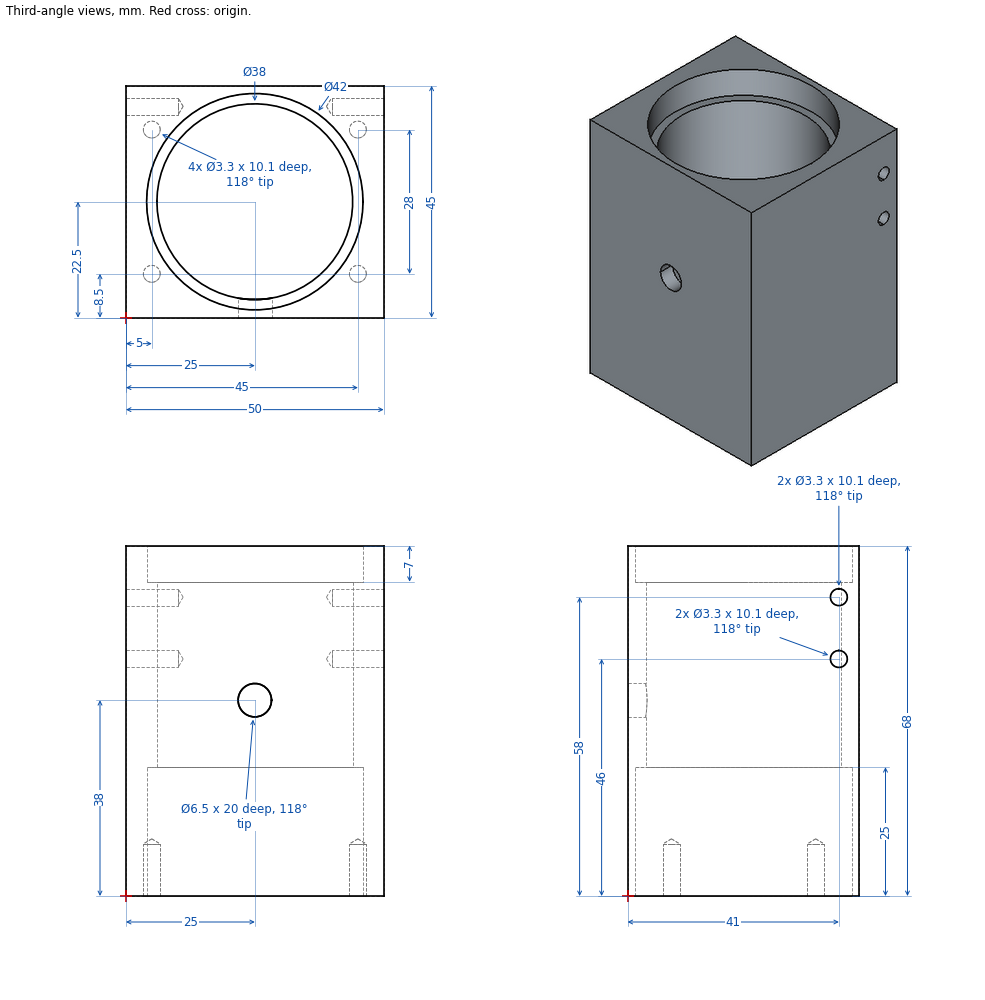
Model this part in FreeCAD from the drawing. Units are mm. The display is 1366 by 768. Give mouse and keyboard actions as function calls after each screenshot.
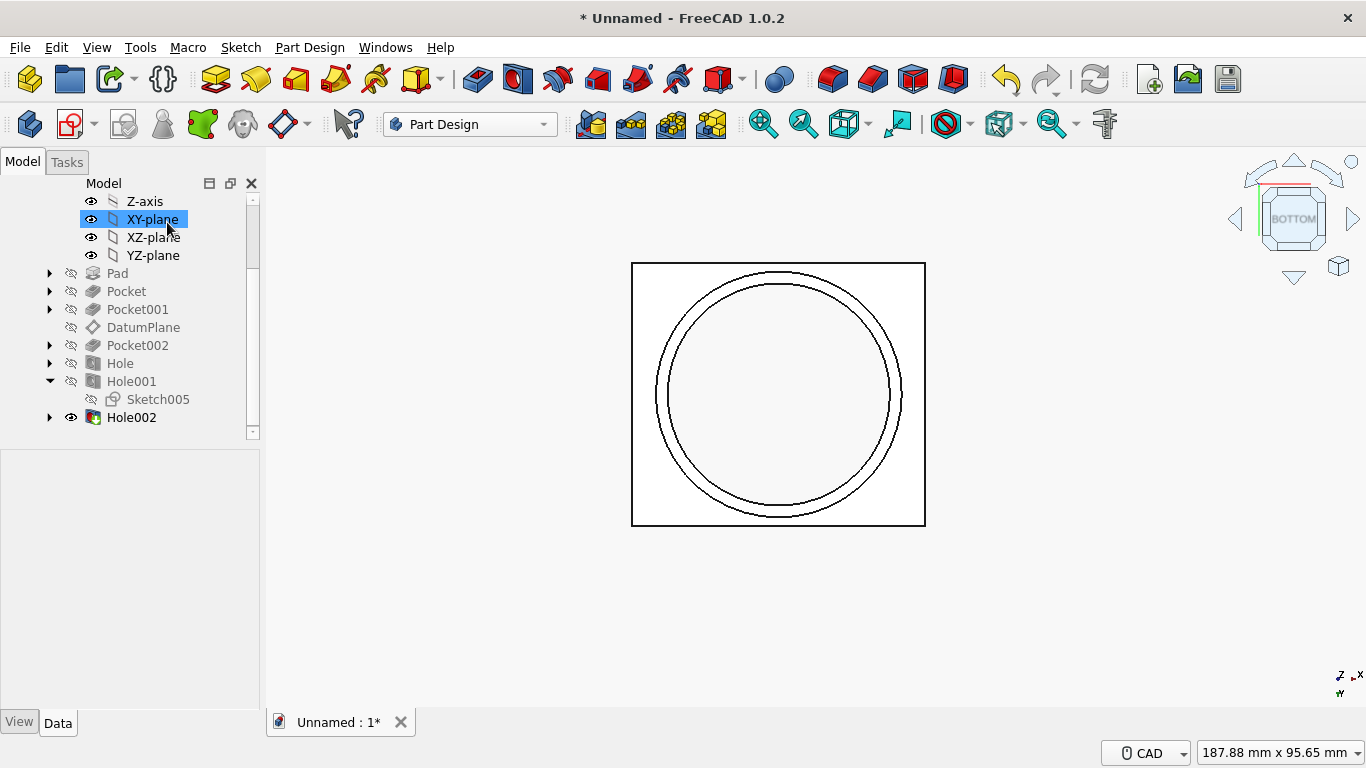
click(653, 469)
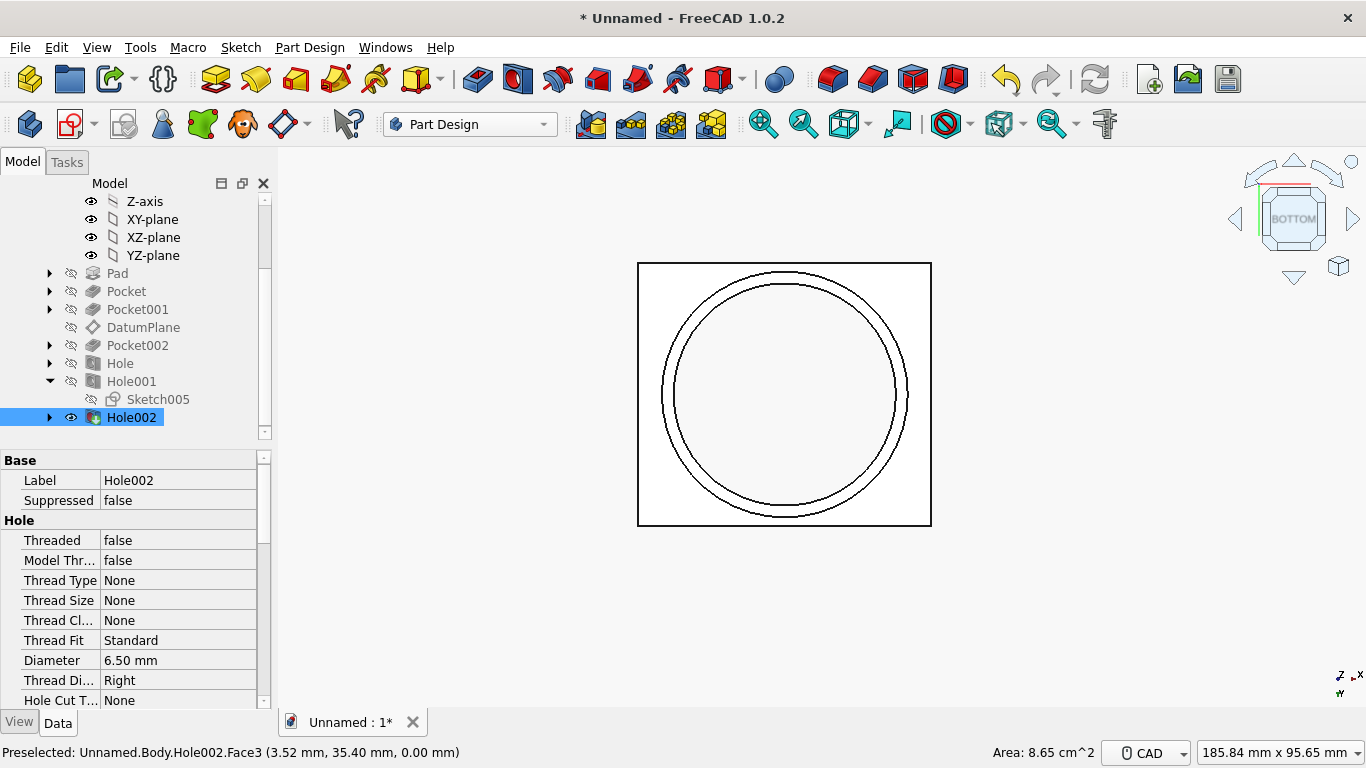
click(70, 124)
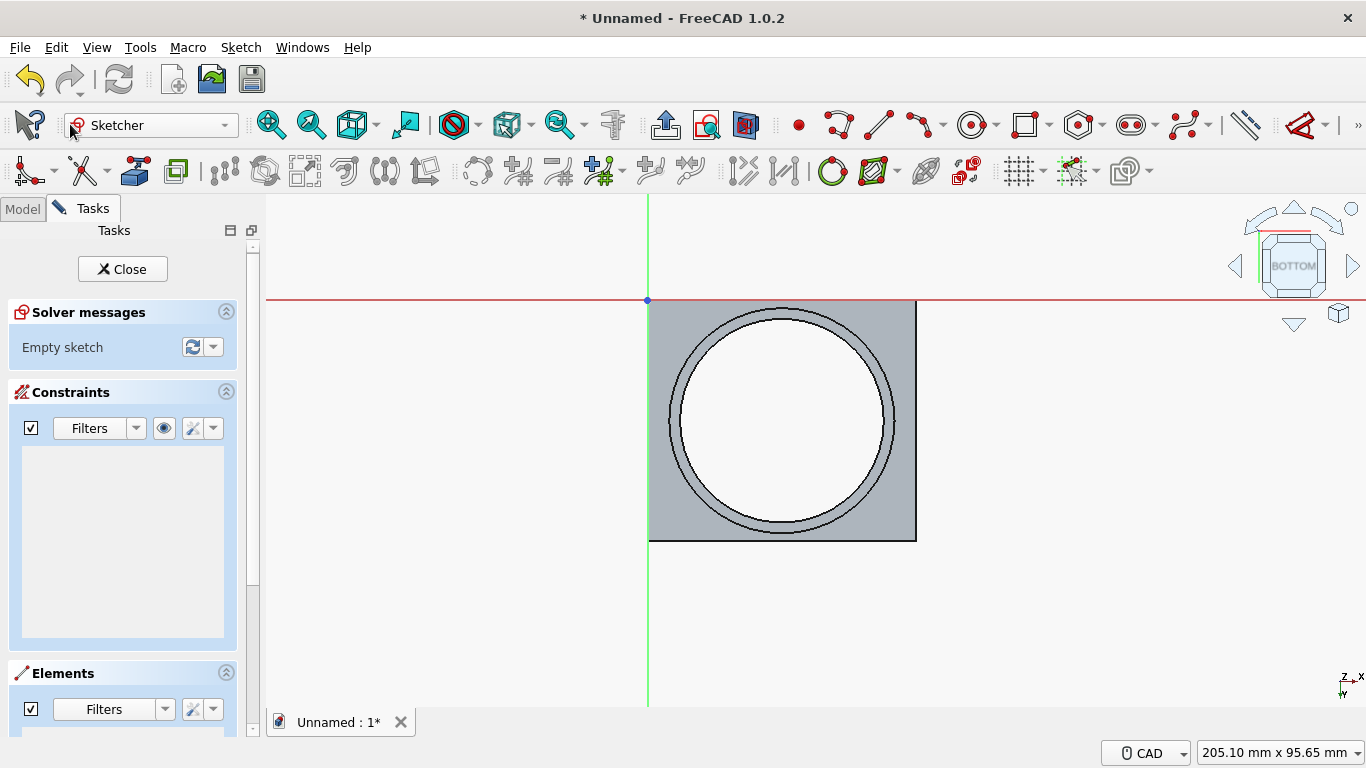
scroll(825, 304, up, 2)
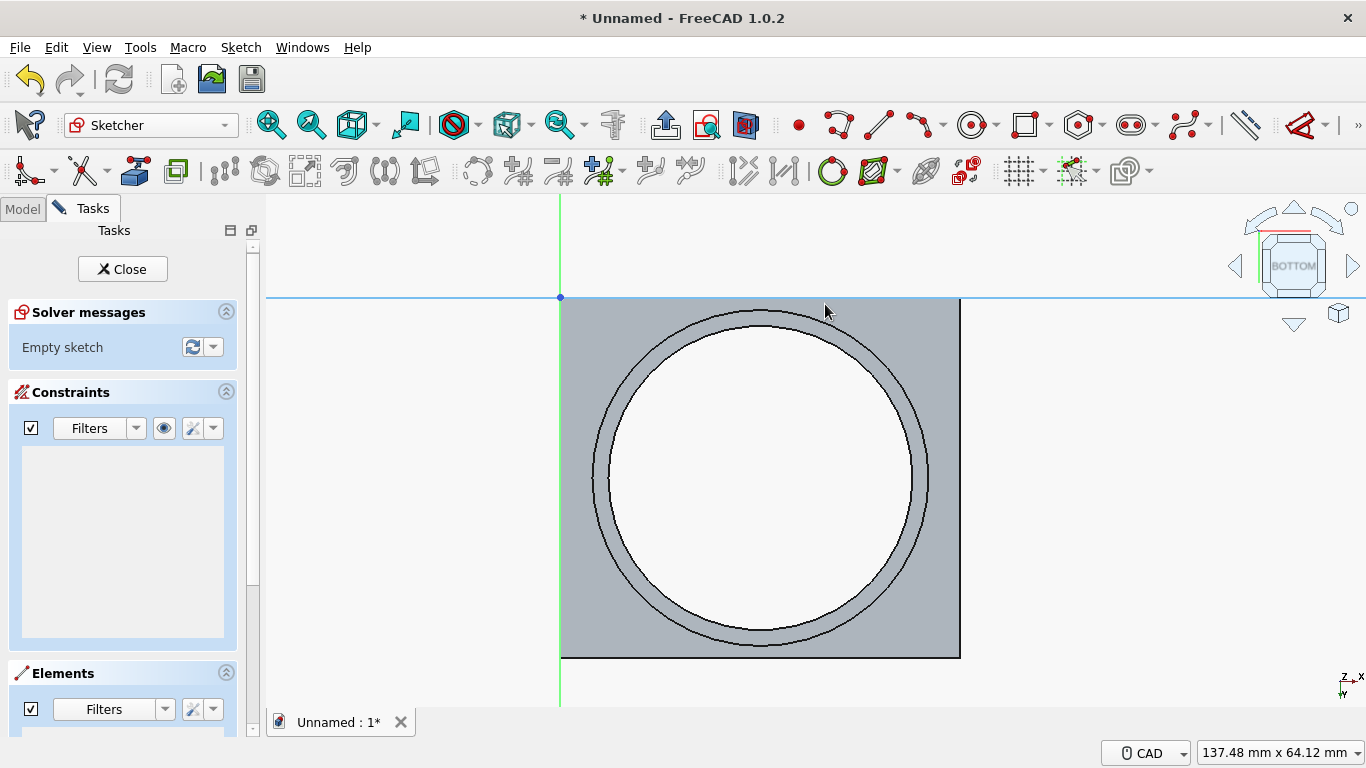
key(g)
key(c)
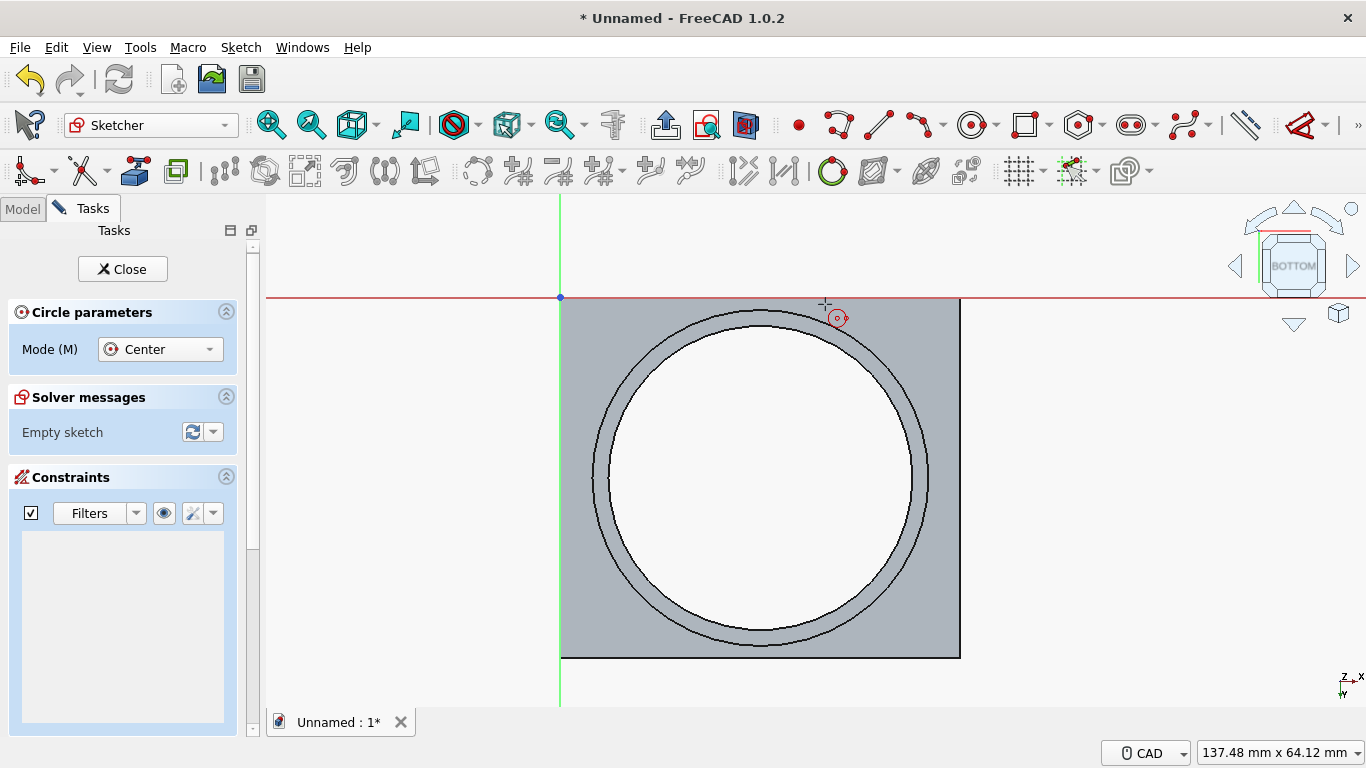
scroll(600, 590, up, 3)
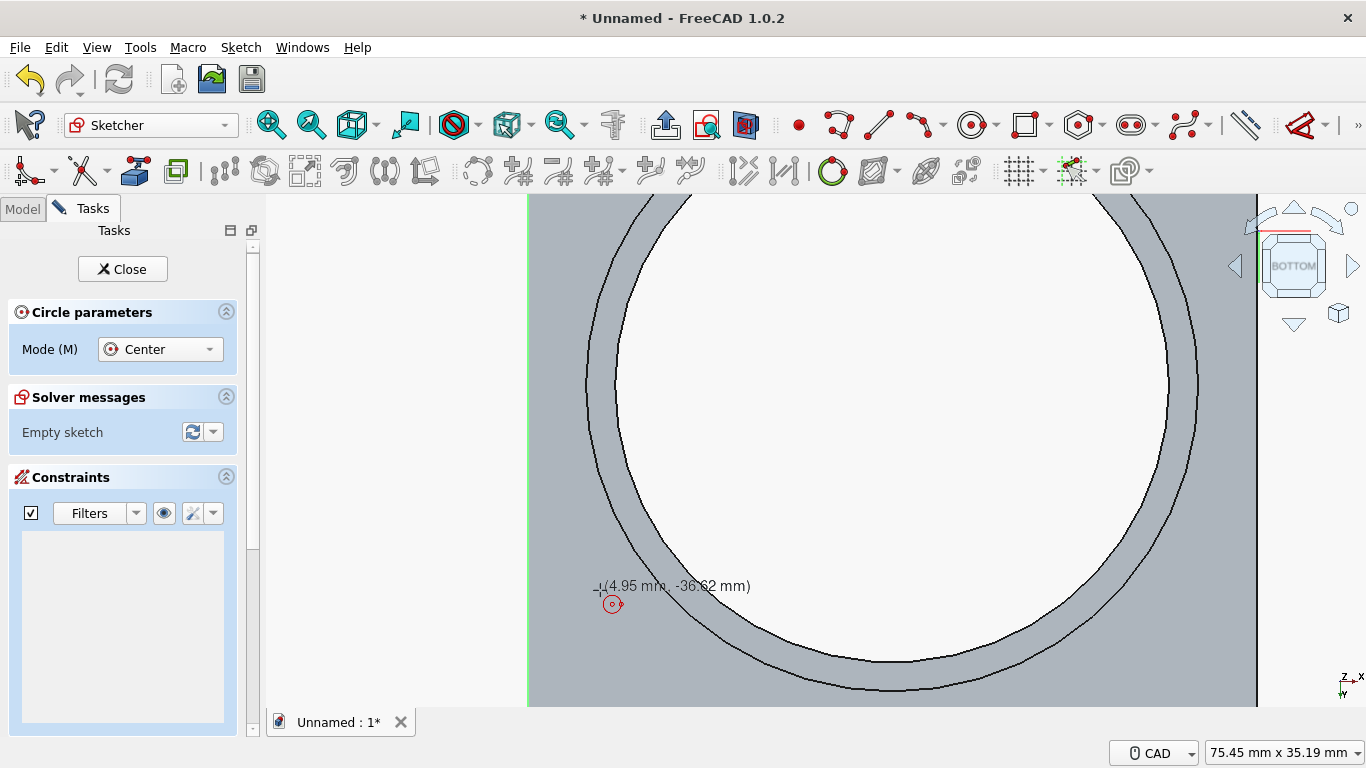
click(601, 589)
move(618, 572)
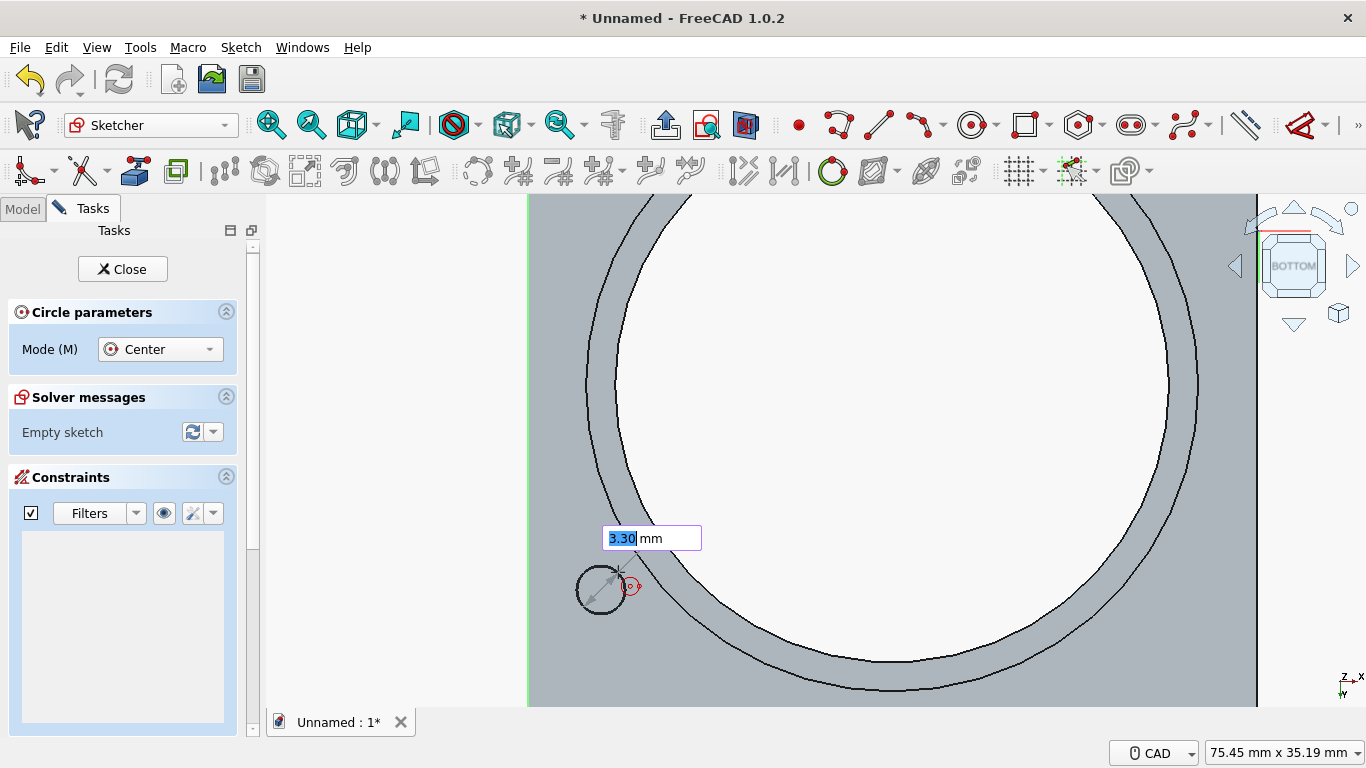
text(3.3)
key(Return)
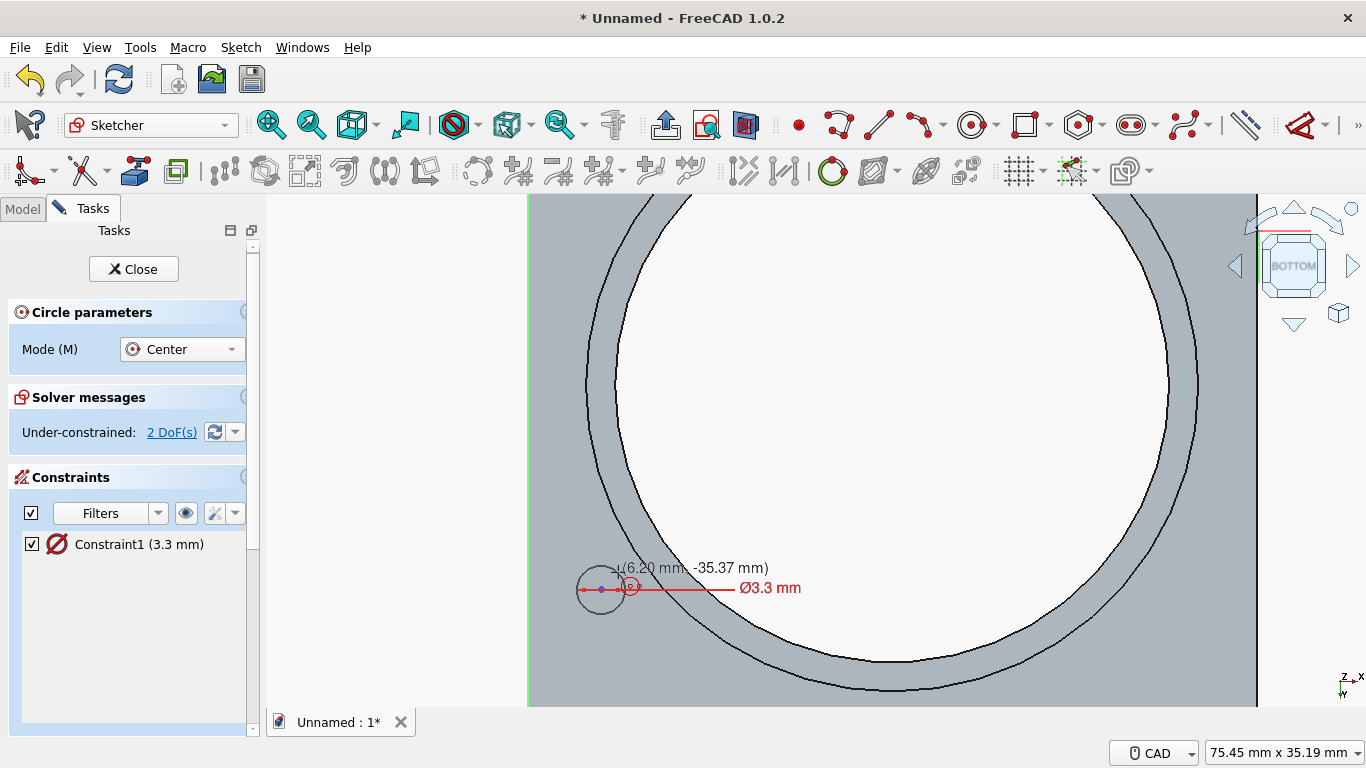
click(1184, 589)
move(1201, 572)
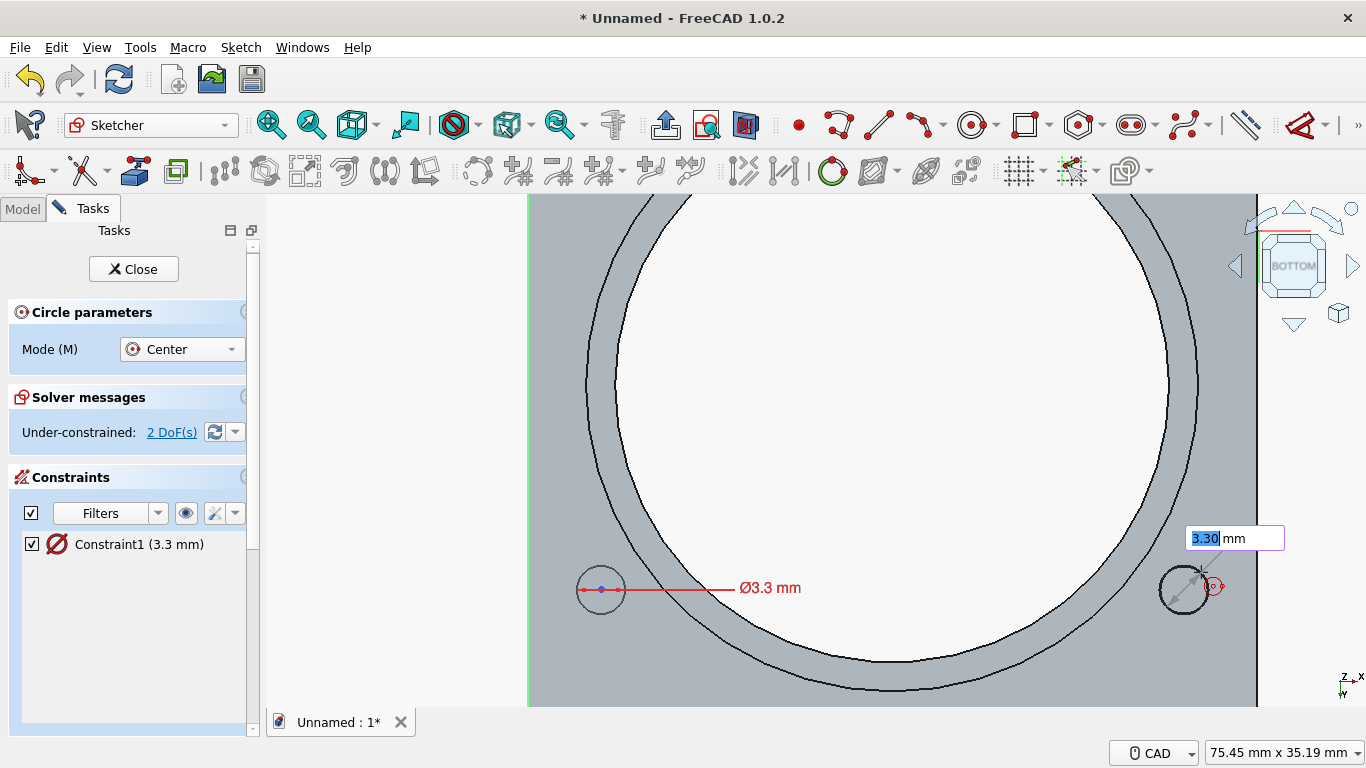
text(3.3)
key(Return)